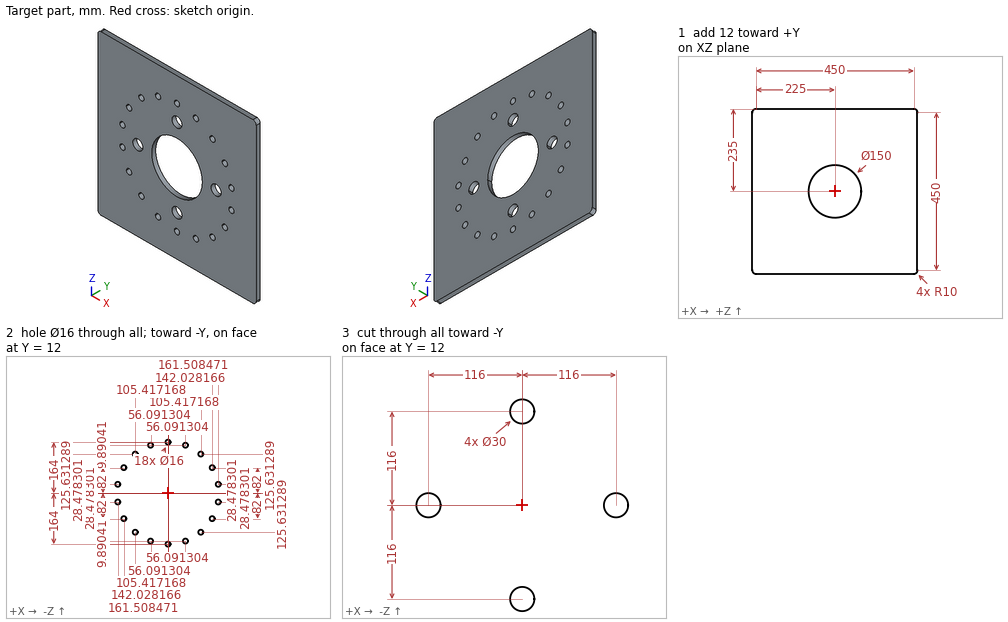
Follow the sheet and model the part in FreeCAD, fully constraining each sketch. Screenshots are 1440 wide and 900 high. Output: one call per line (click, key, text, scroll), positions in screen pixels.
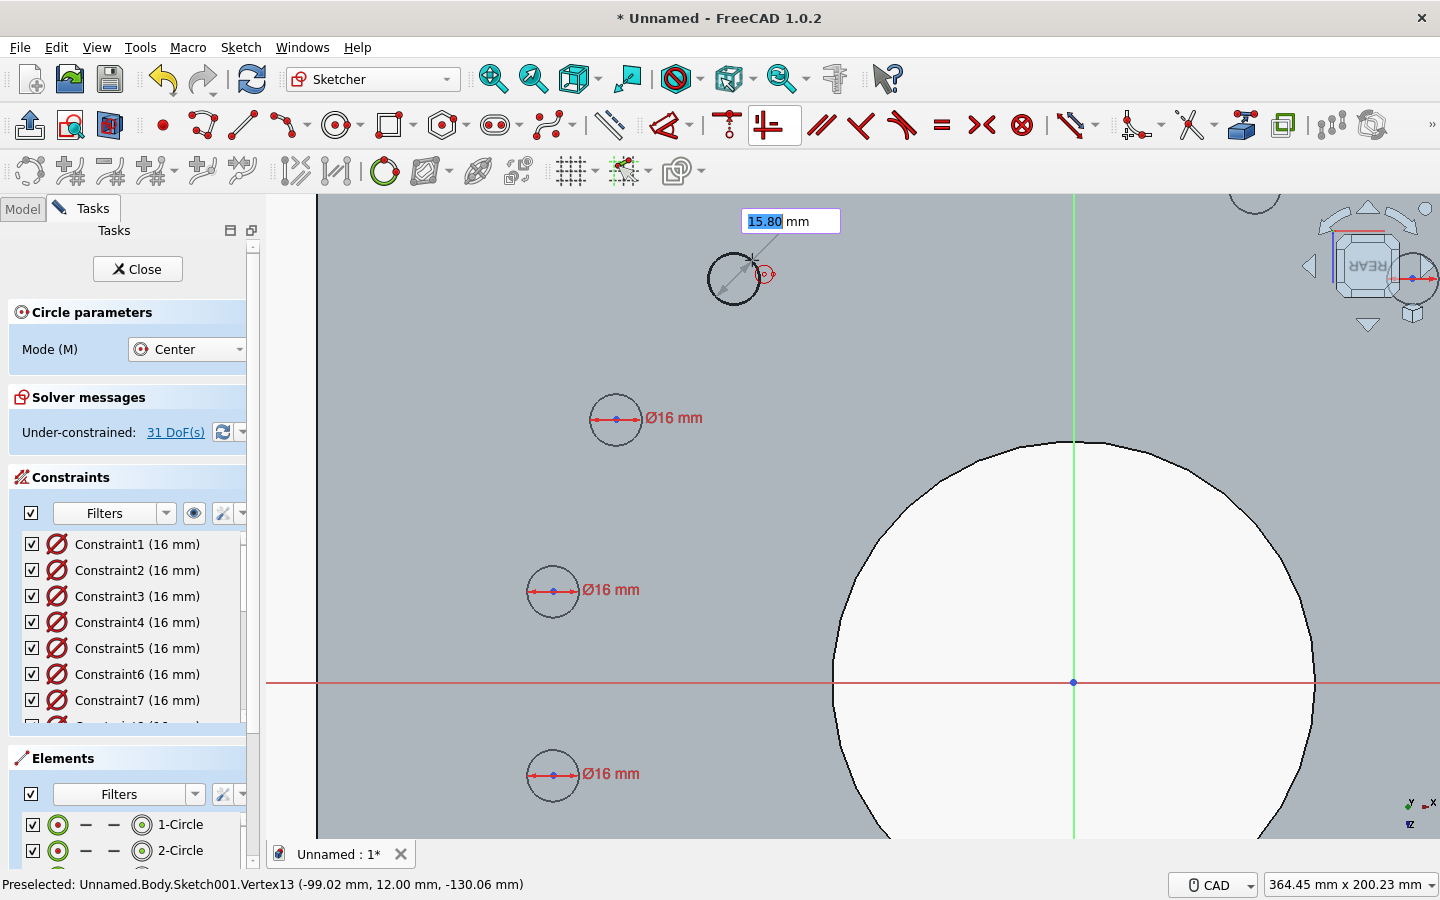
text(16)
key(Return)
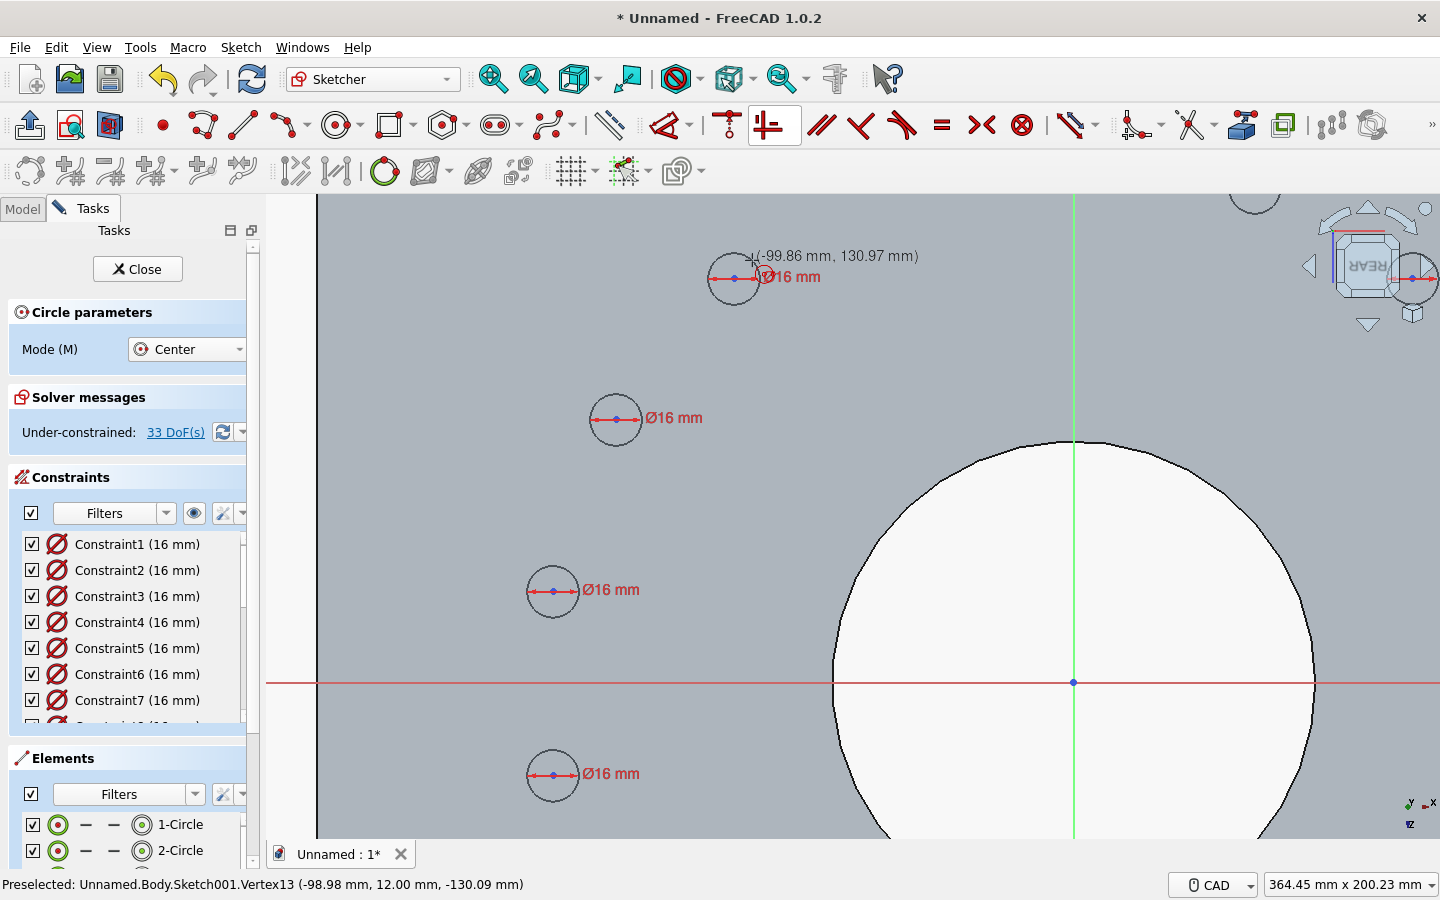
scroll(616, 420, down, 5)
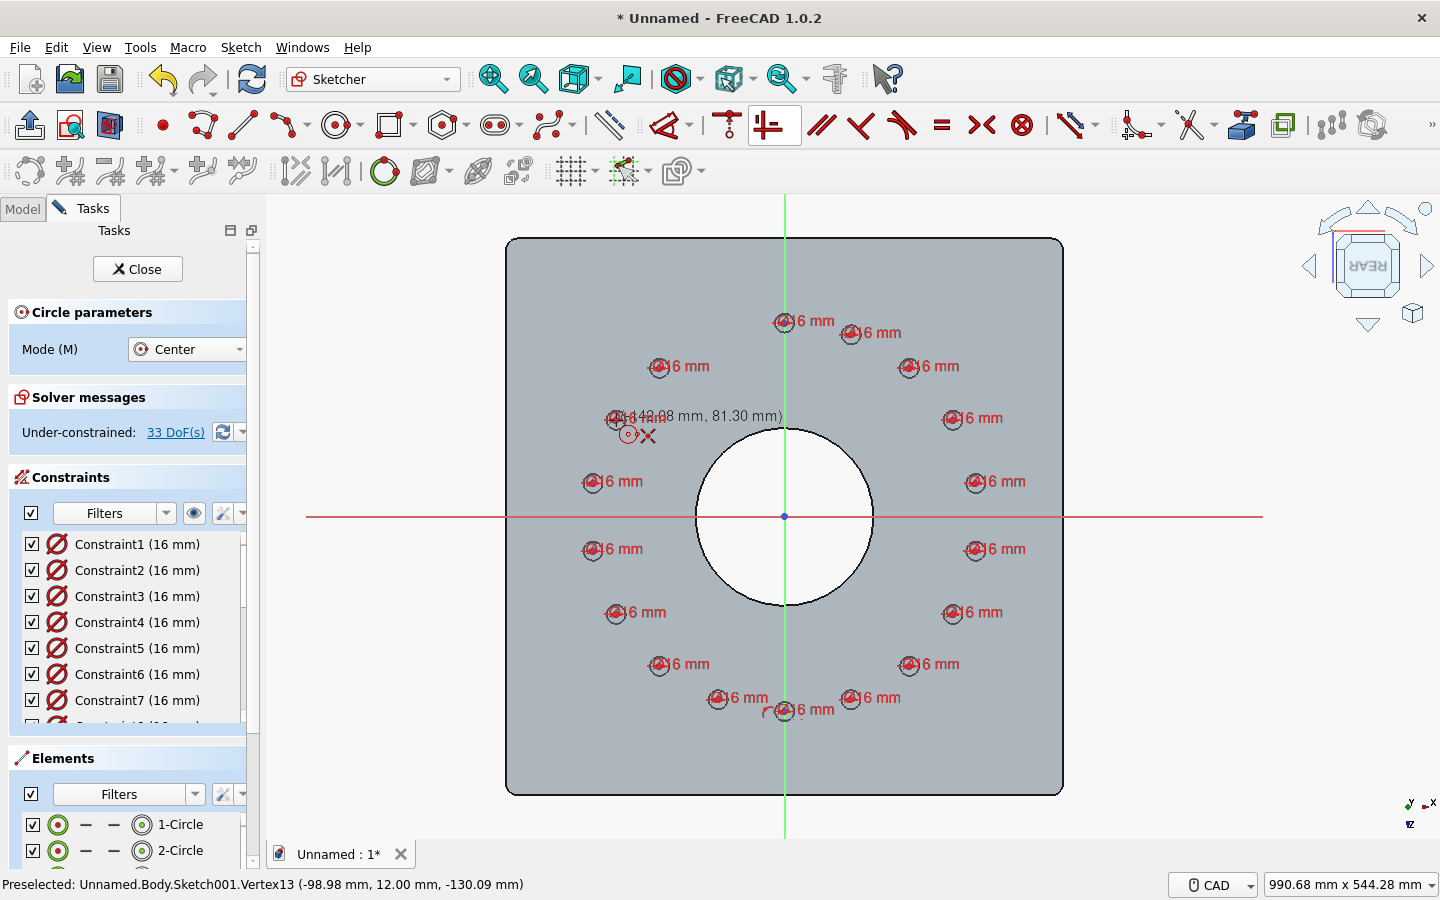
scroll(718, 334, up, 5)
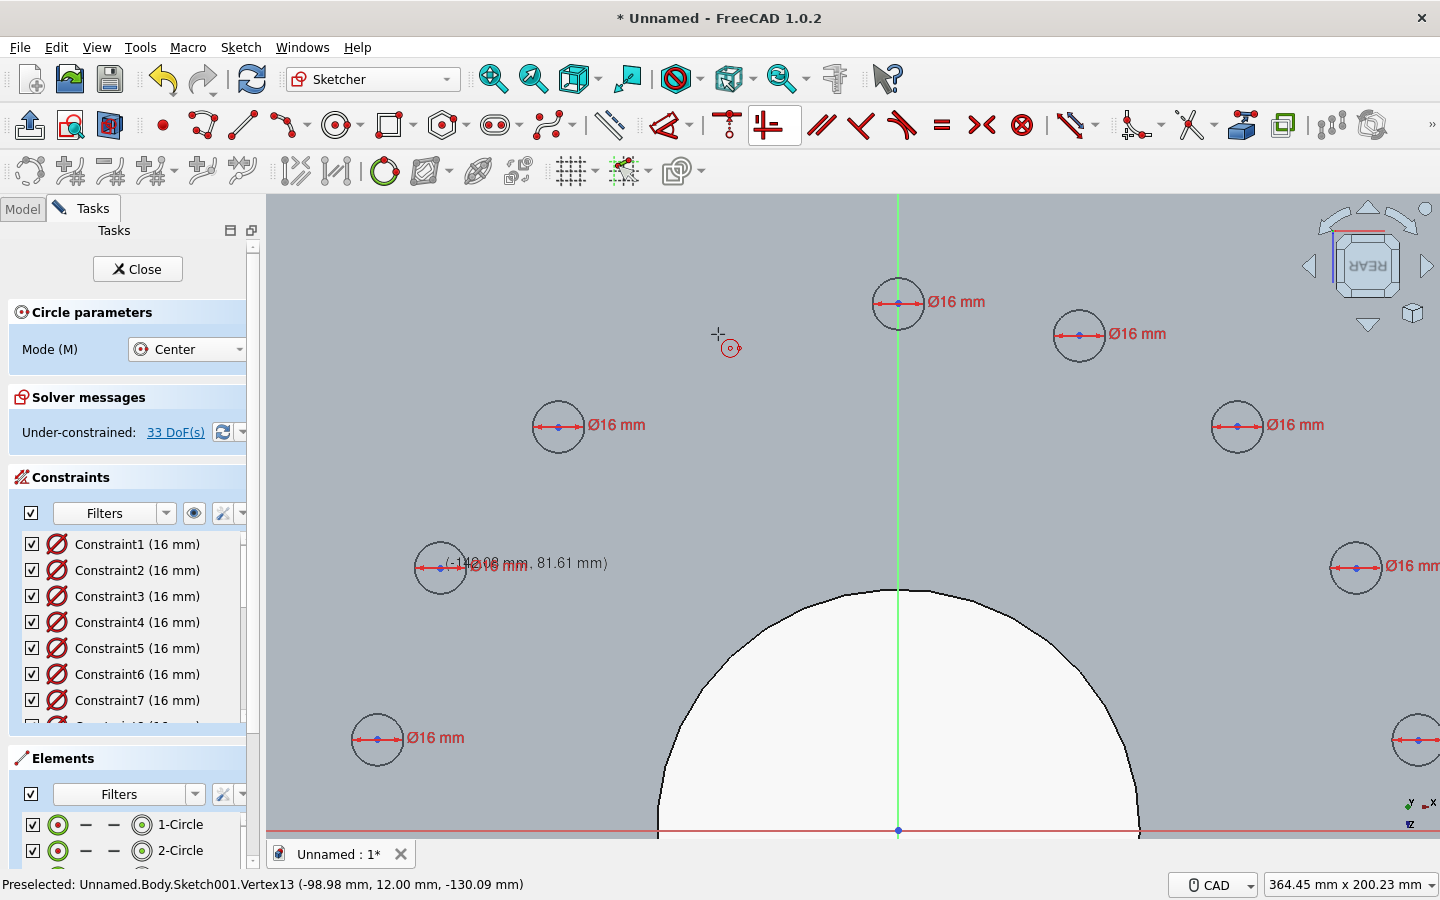
click(718, 334)
move(736, 316)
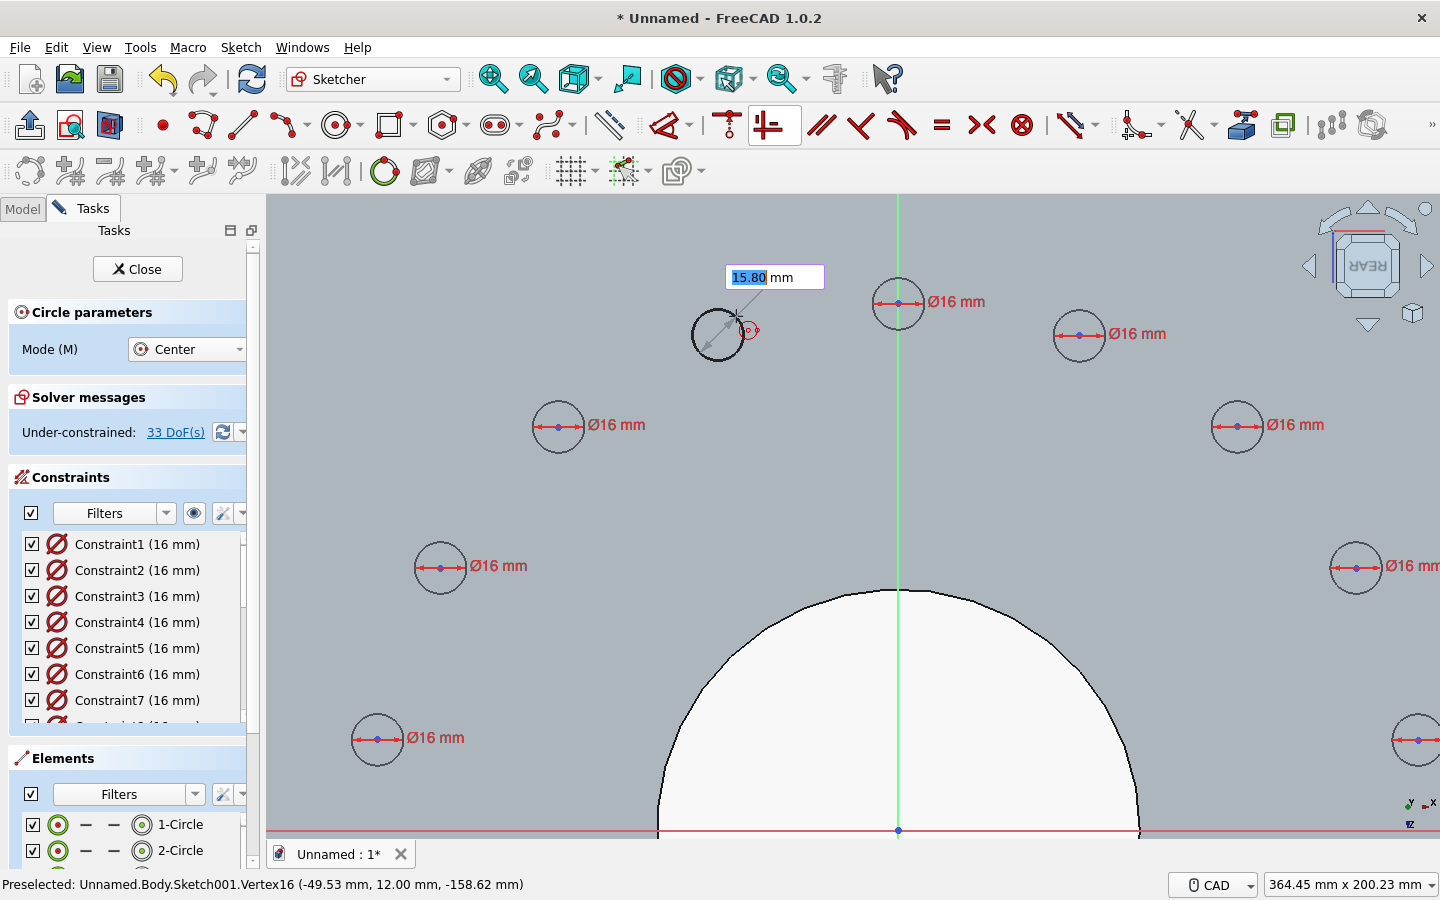
text(16)
key(Return)
key(Escape)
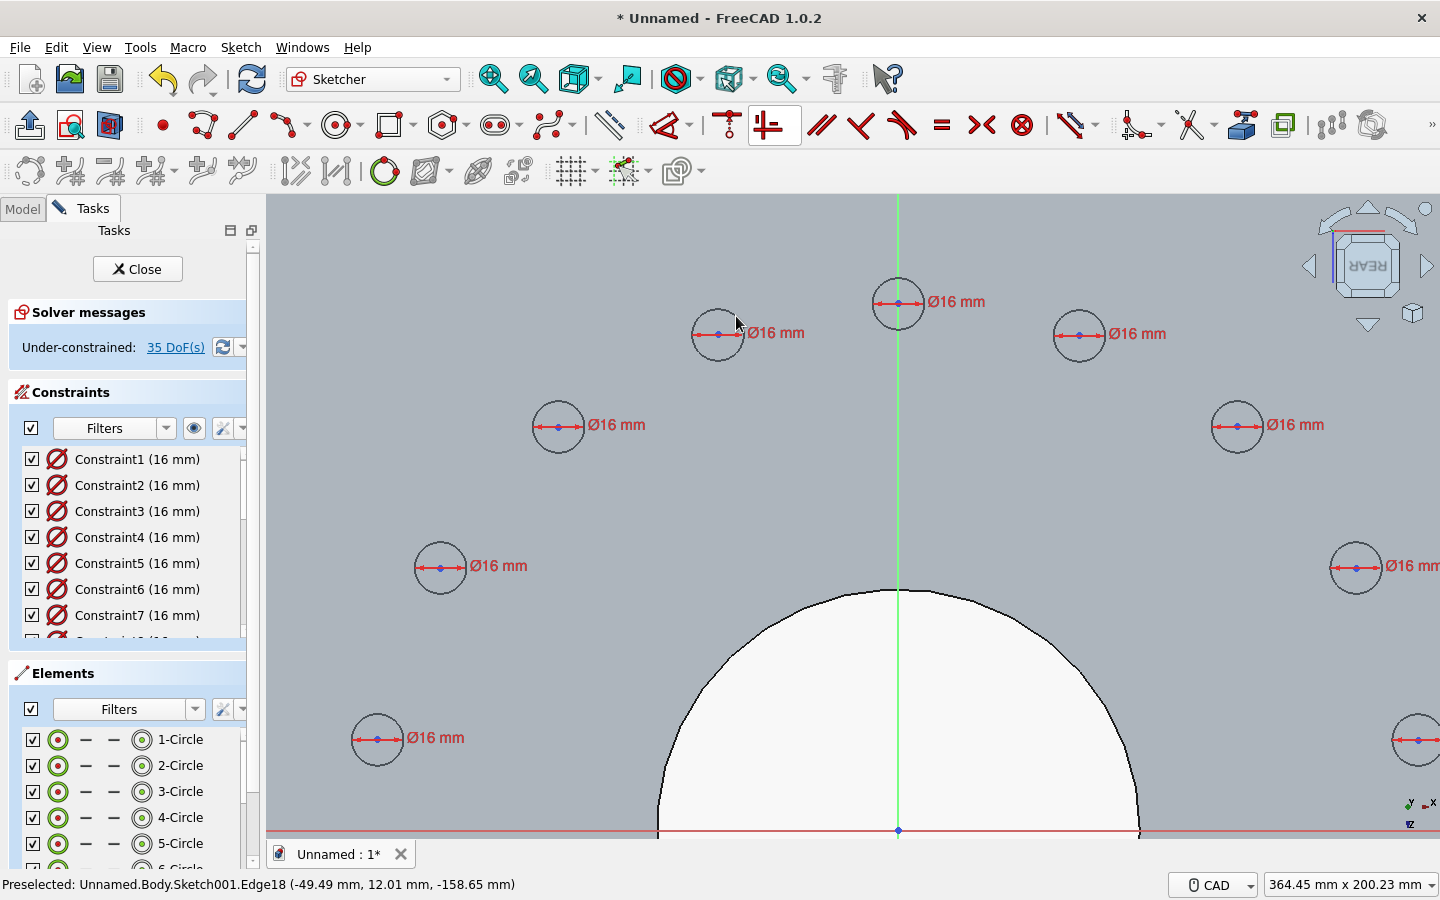
click(898, 304)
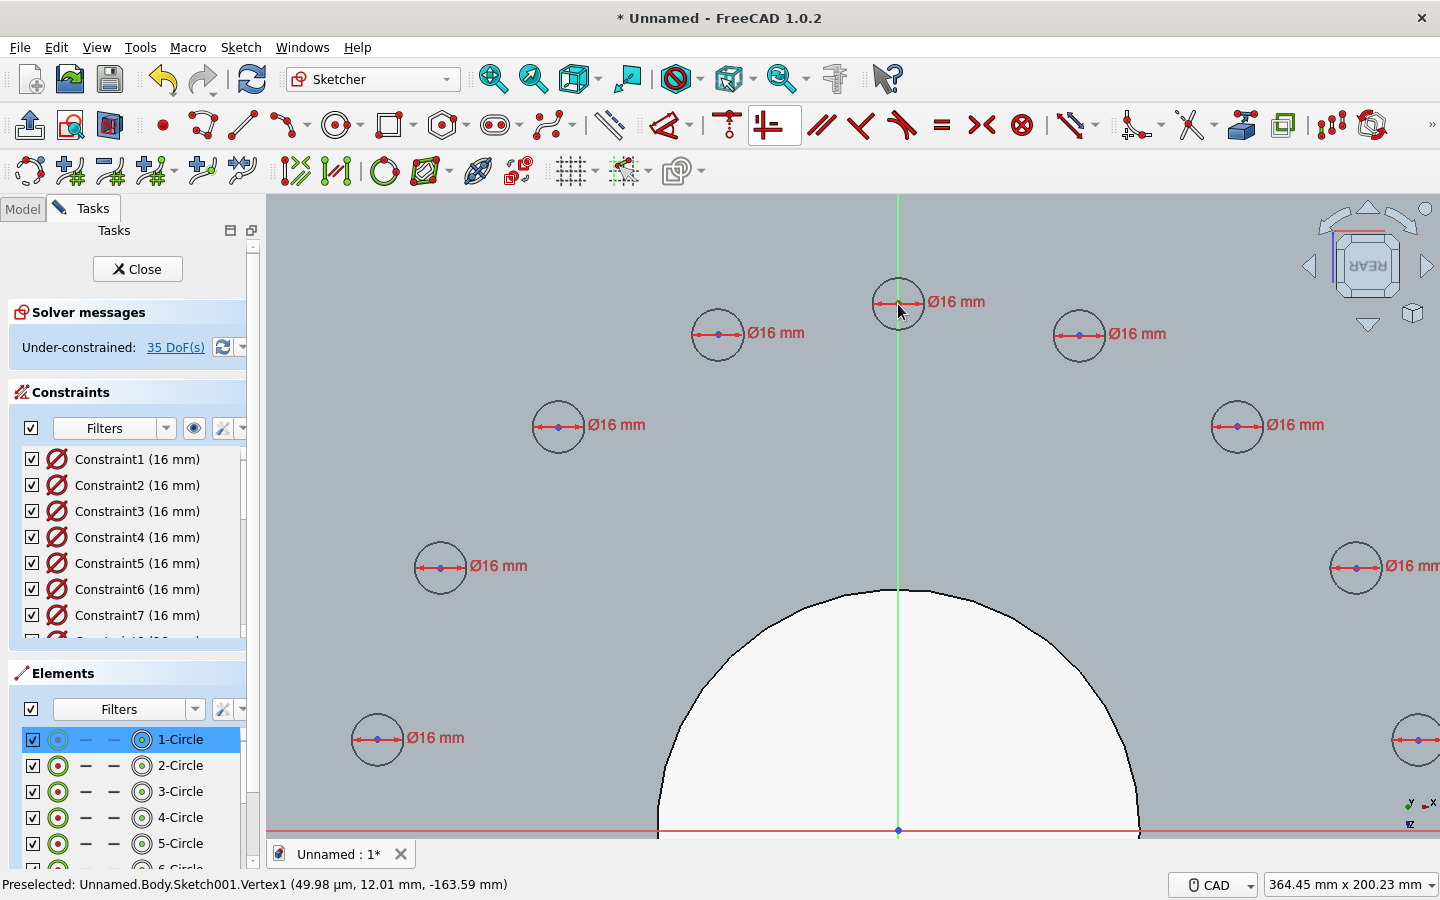
click(898, 769)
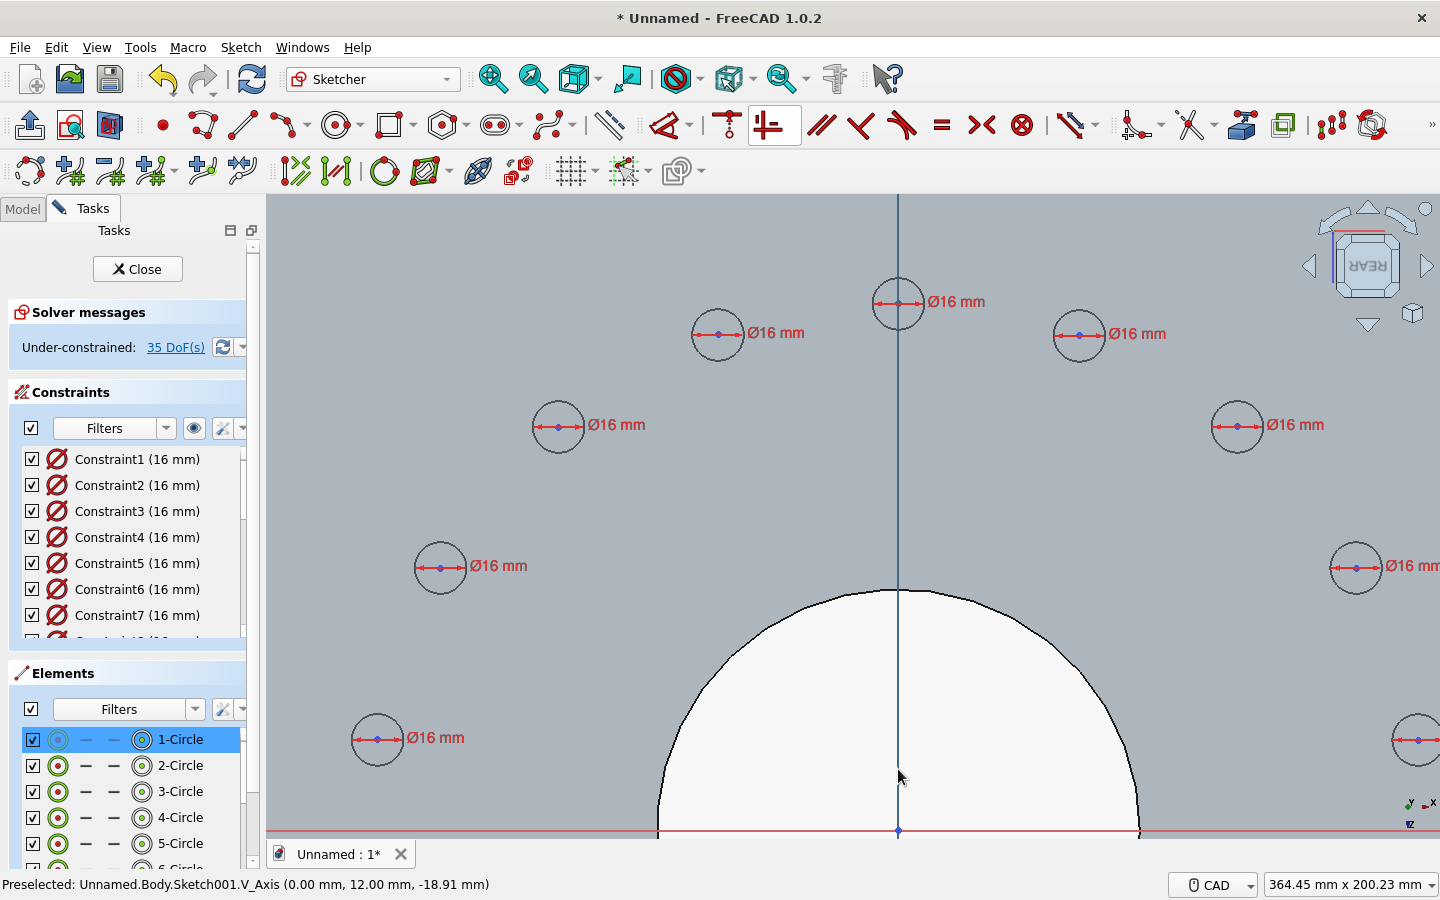
key(c)